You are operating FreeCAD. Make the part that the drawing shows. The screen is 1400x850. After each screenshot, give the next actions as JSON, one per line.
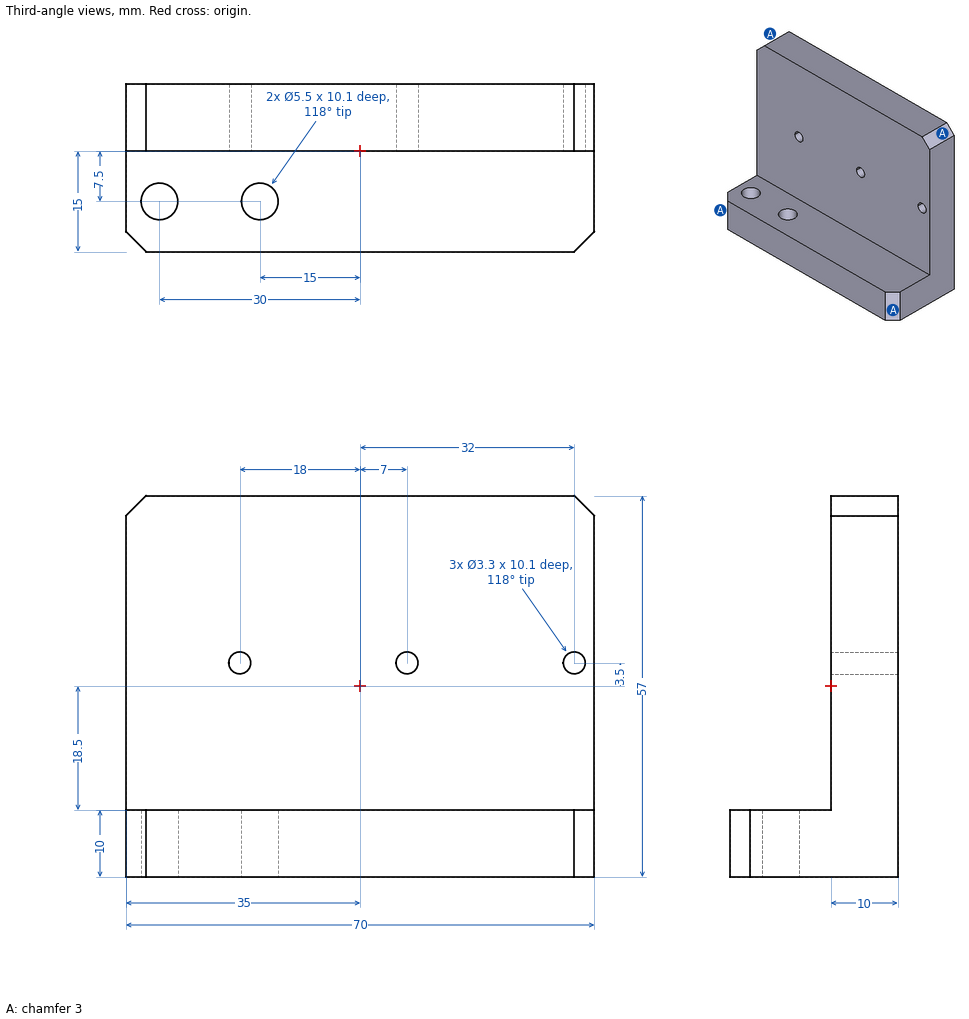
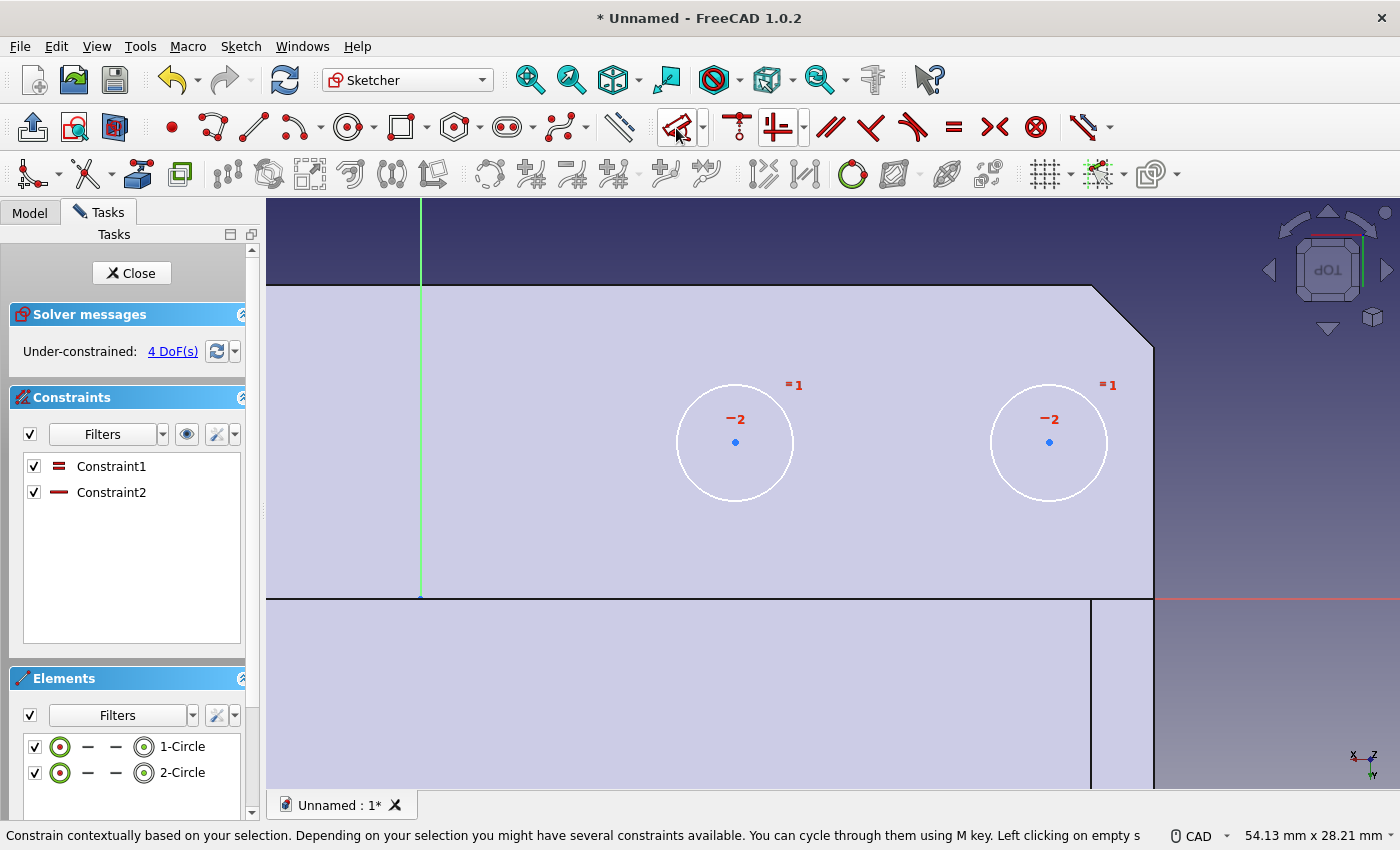
{"action": "left_click", "coordinate": [776, 402]}
{"action": "left_click", "coordinate": [799, 379]}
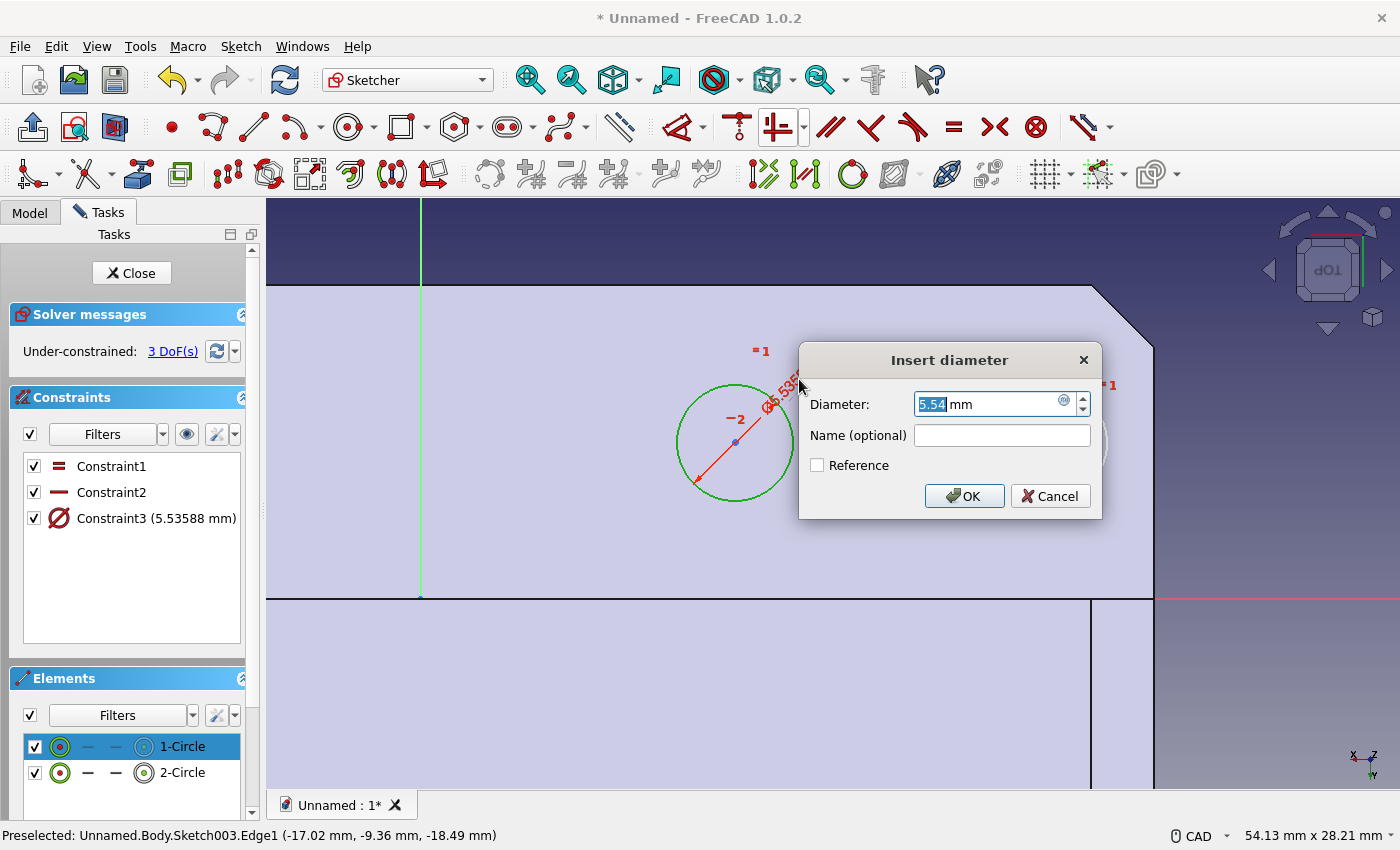
{"action": "type", "text": "5.5"}
{"action": "key", "text": "Return"}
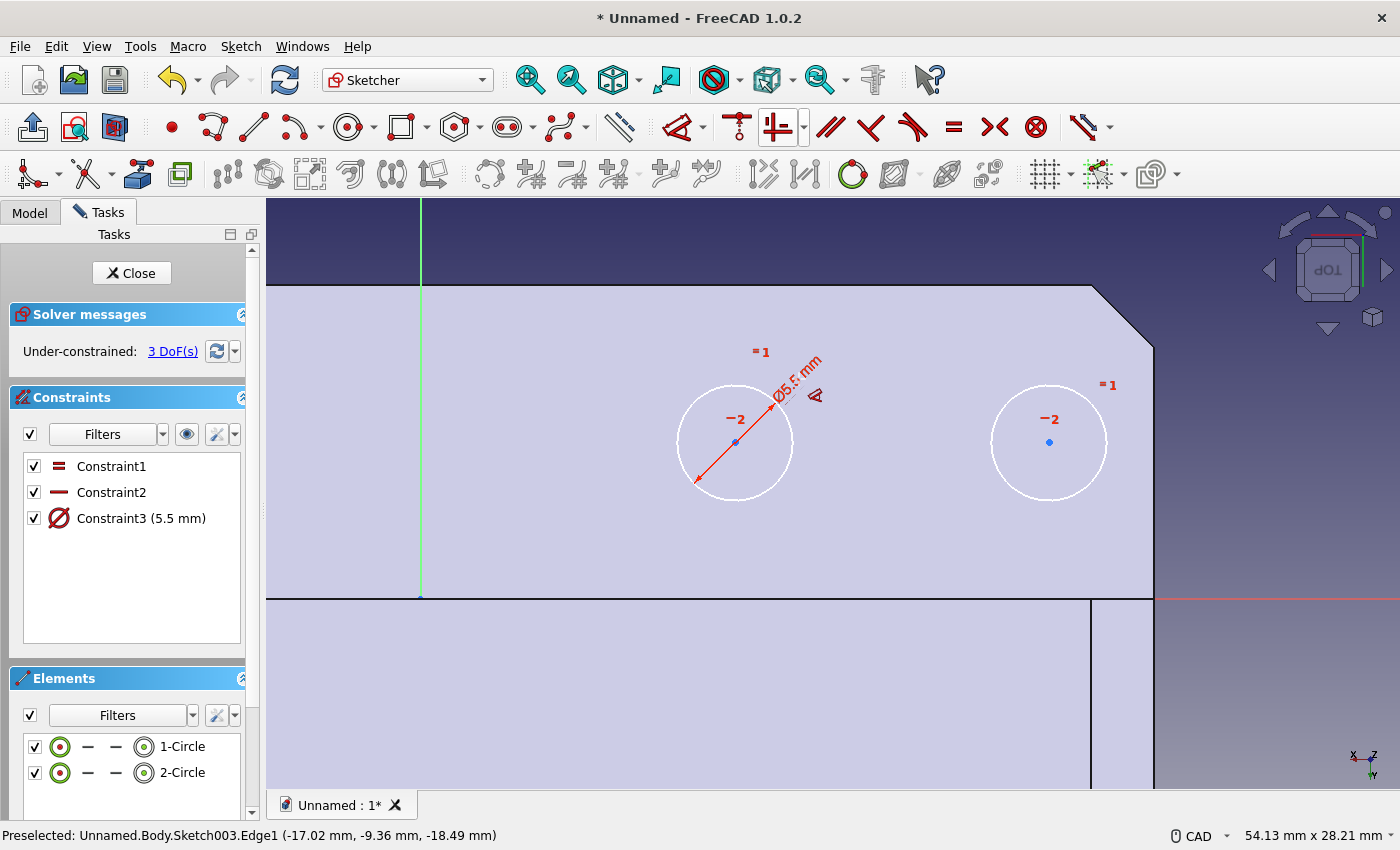
{"action": "left_click", "coordinate": [735, 443]}
{"action": "left_click", "coordinate": [578, 633]}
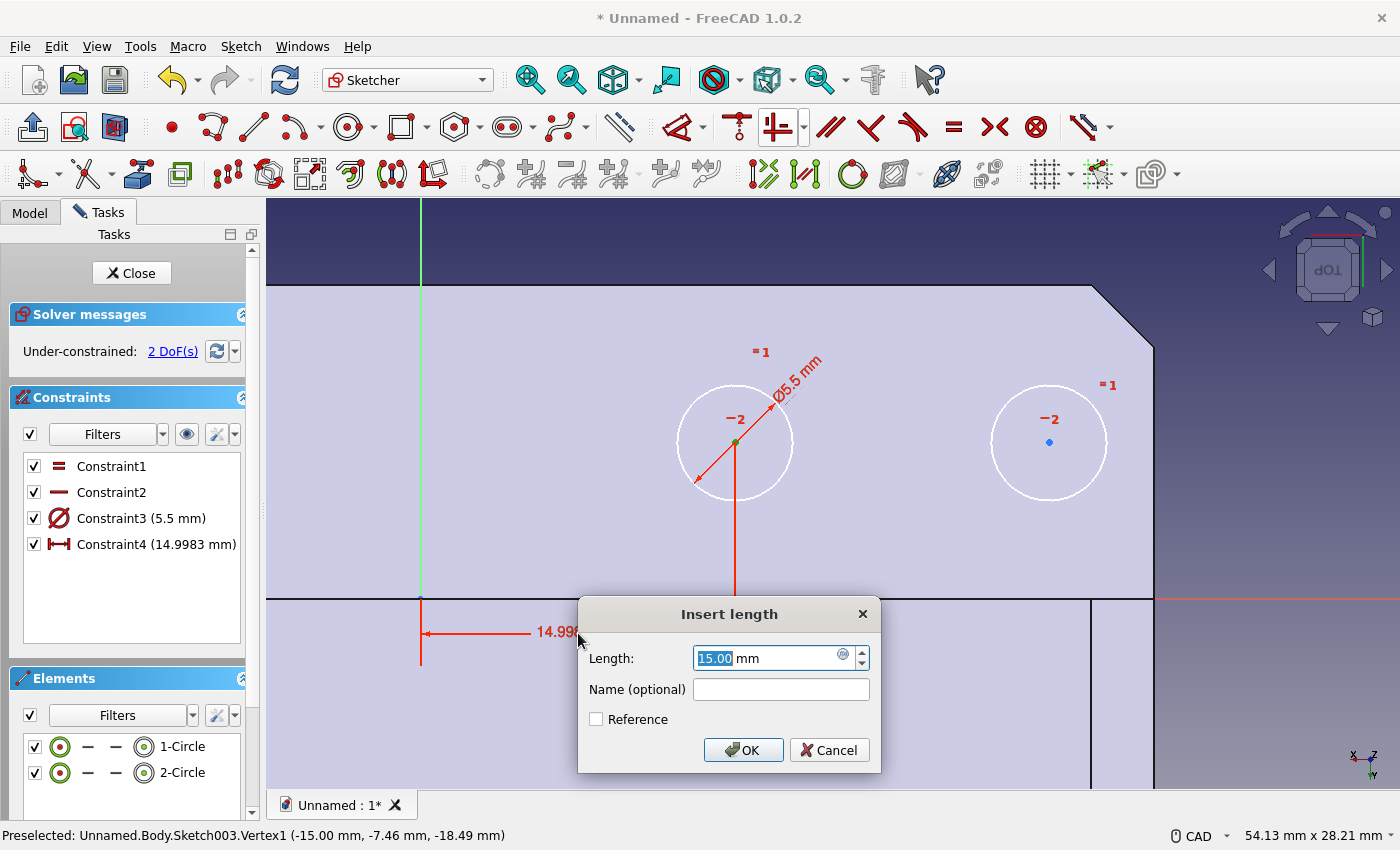
{"action": "type", "text": "15"}
{"action": "key", "text": "Return"}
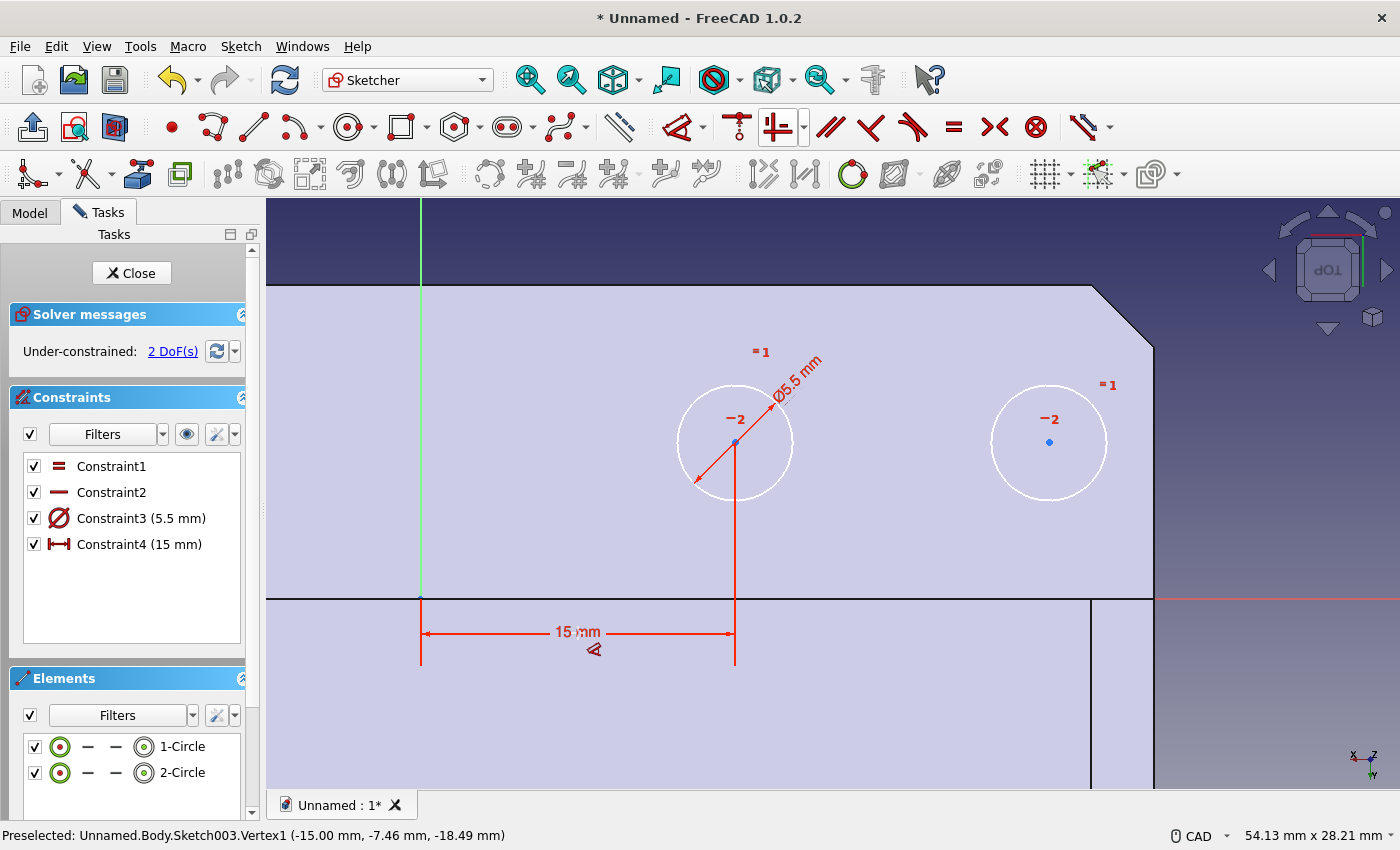
{"action": "left_click", "coordinate": [1049, 443]}
{"action": "left_click", "coordinate": [735, 633]}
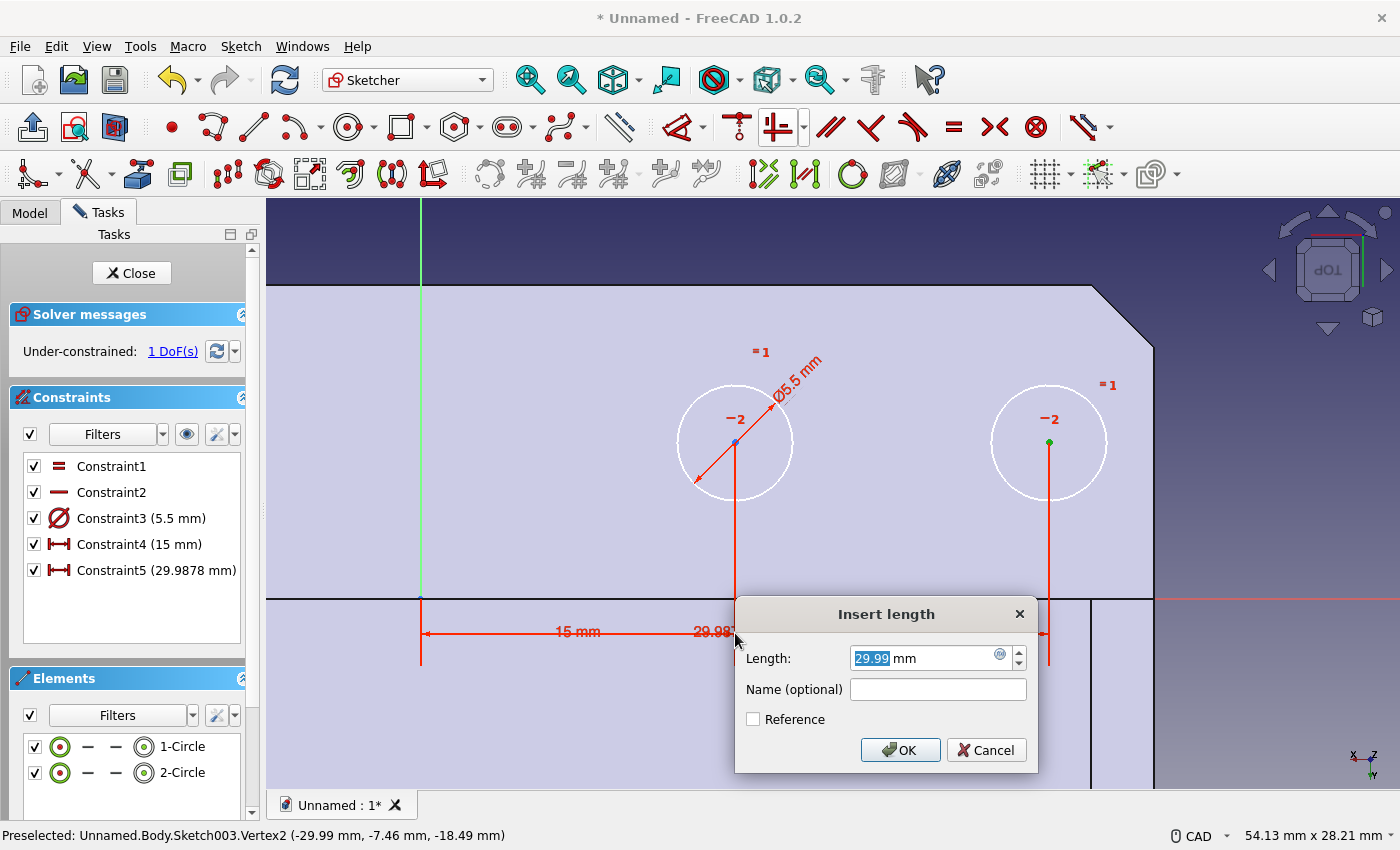
{"action": "type", "text": "30"}
{"action": "key", "text": "Return"}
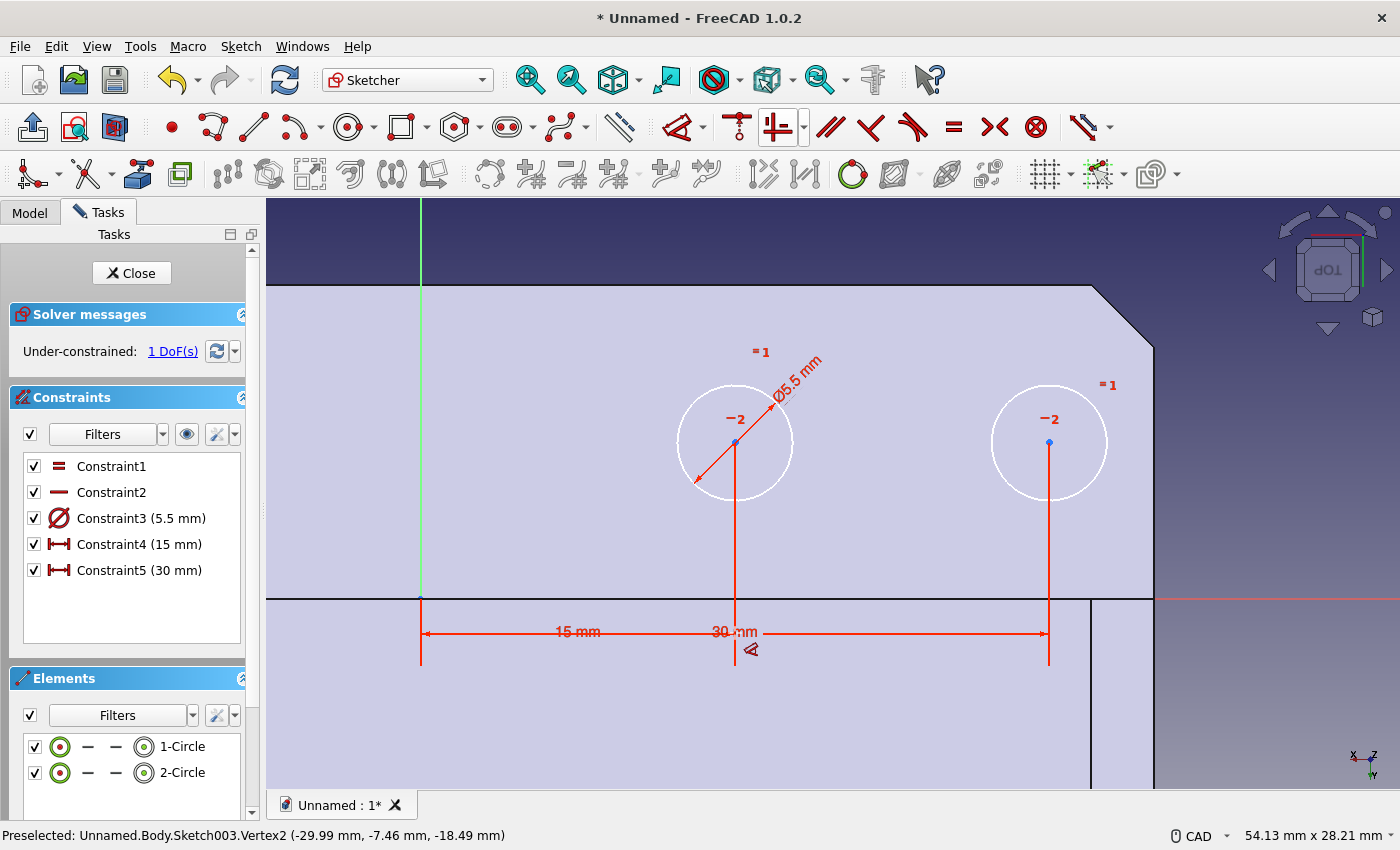
{"action": "left_click", "coordinate": [735, 443]}
{"action": "left_click", "coordinate": [387, 521]}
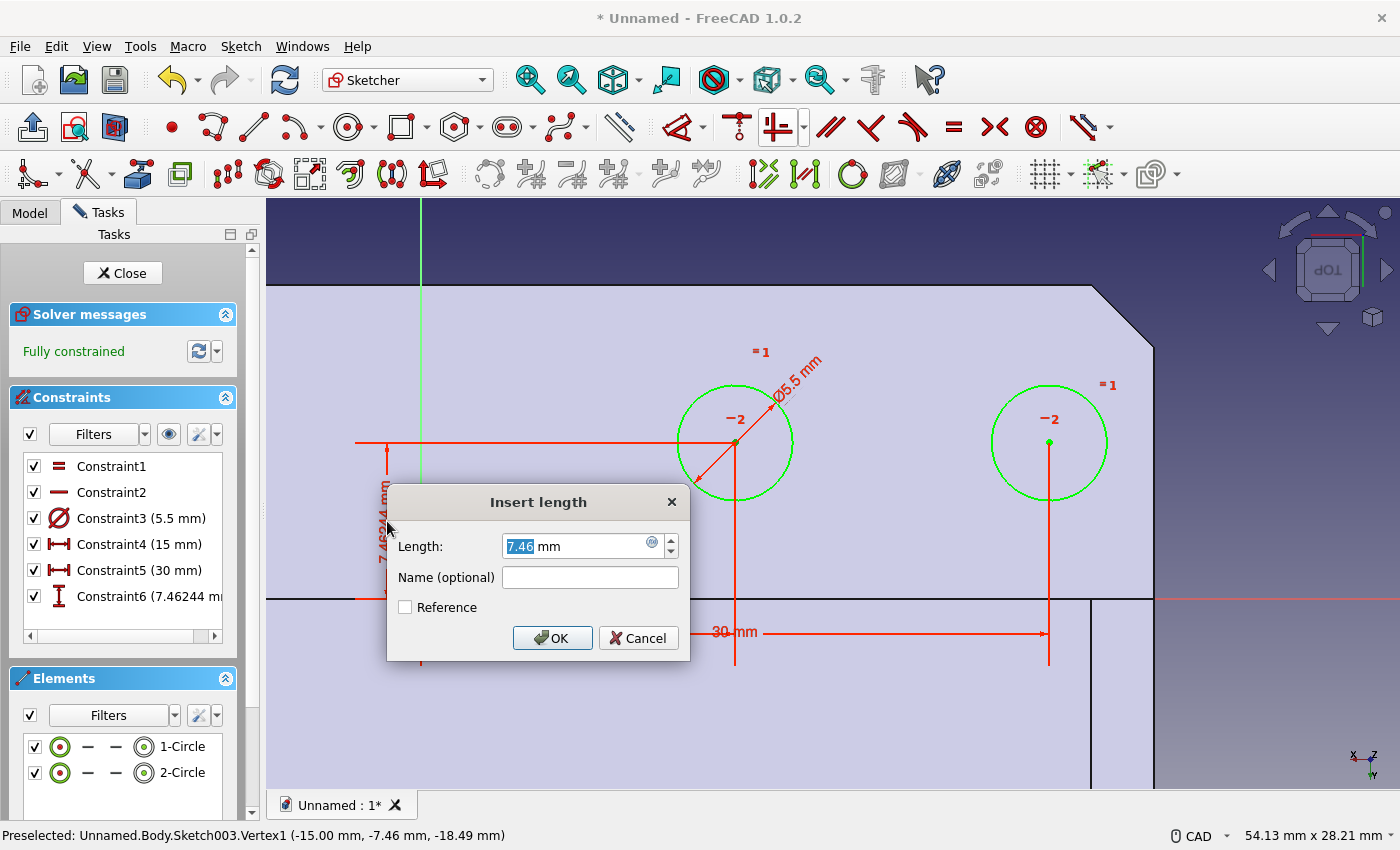
{"action": "type", "text": "7.5"}
{"action": "key", "text": "Return"}
{"action": "key", "text": "Escape"}